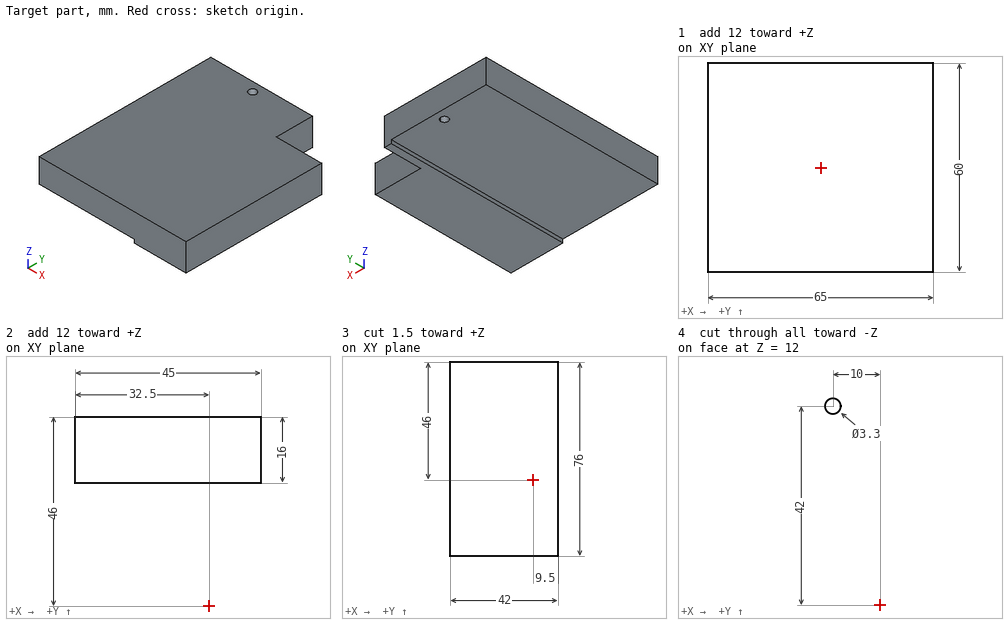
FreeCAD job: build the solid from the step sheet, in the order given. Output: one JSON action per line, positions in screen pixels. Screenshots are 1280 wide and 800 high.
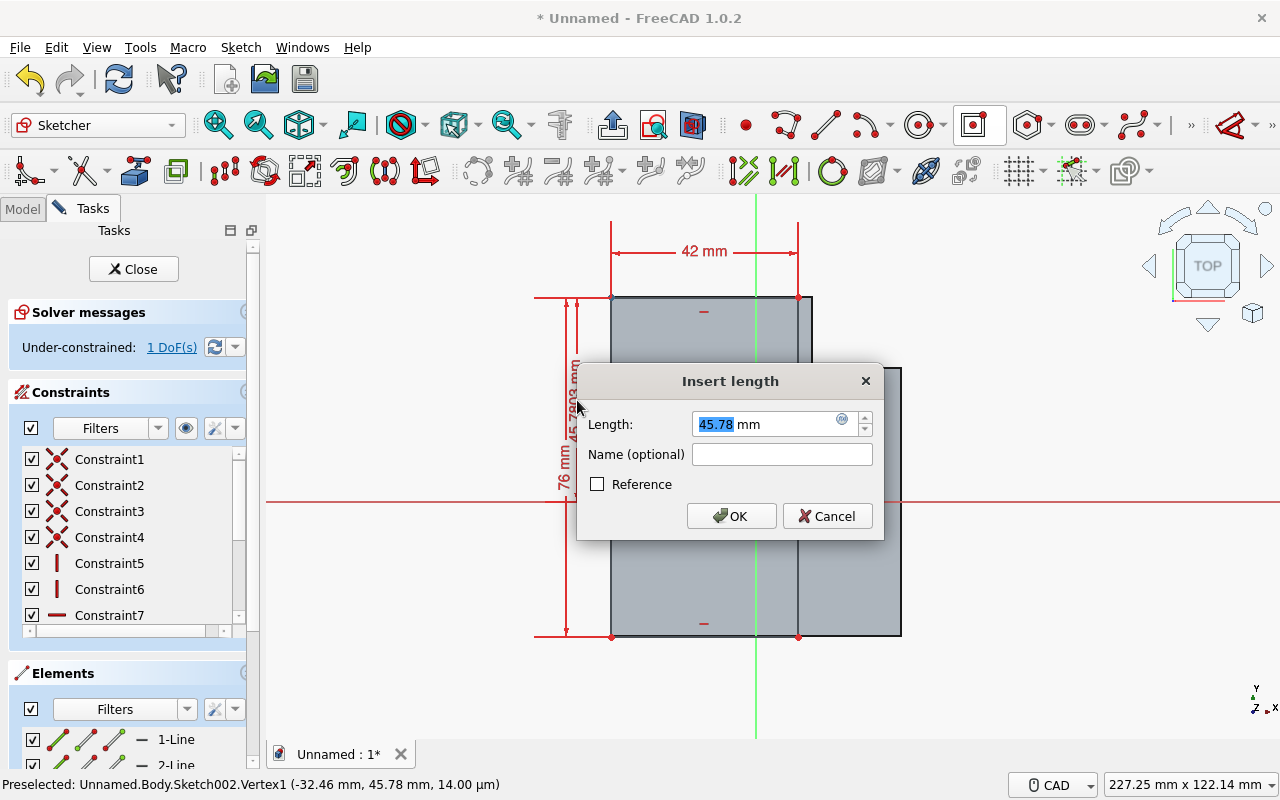
{"action": "type", "text": "46"}
{"action": "key", "text": "Return"}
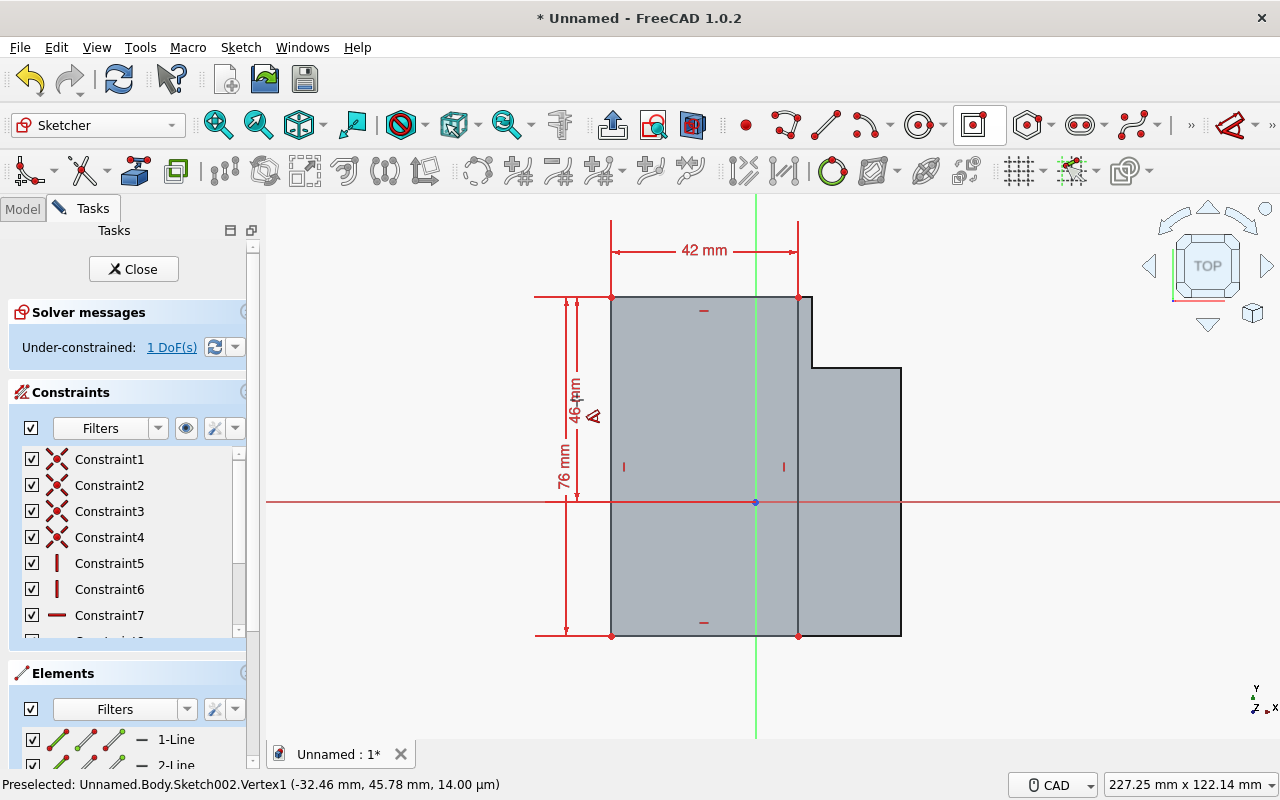
{"action": "left_click", "coordinate": [798, 636]}
{"action": "left_click", "coordinate": [777, 670]}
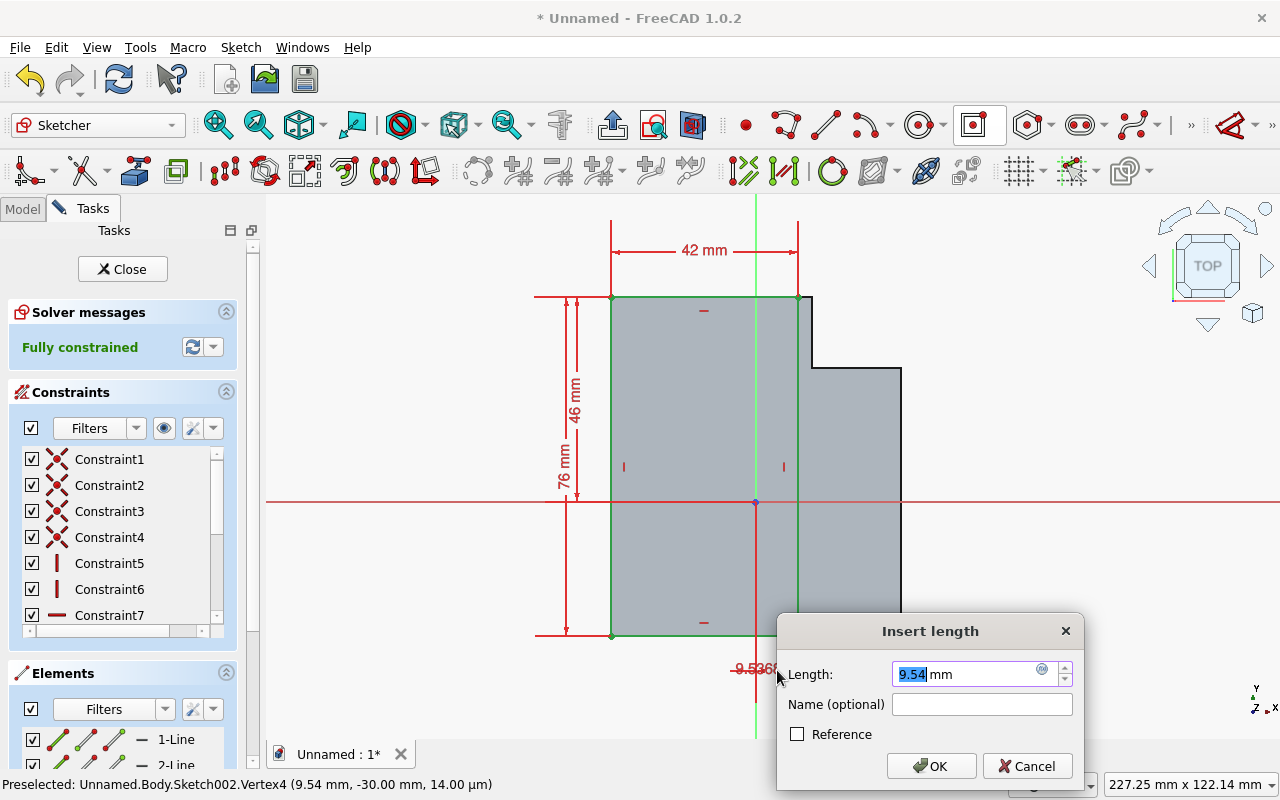
{"action": "type", "text": "9.5"}
{"action": "key", "text": "Return"}
{"action": "key", "text": "Escape"}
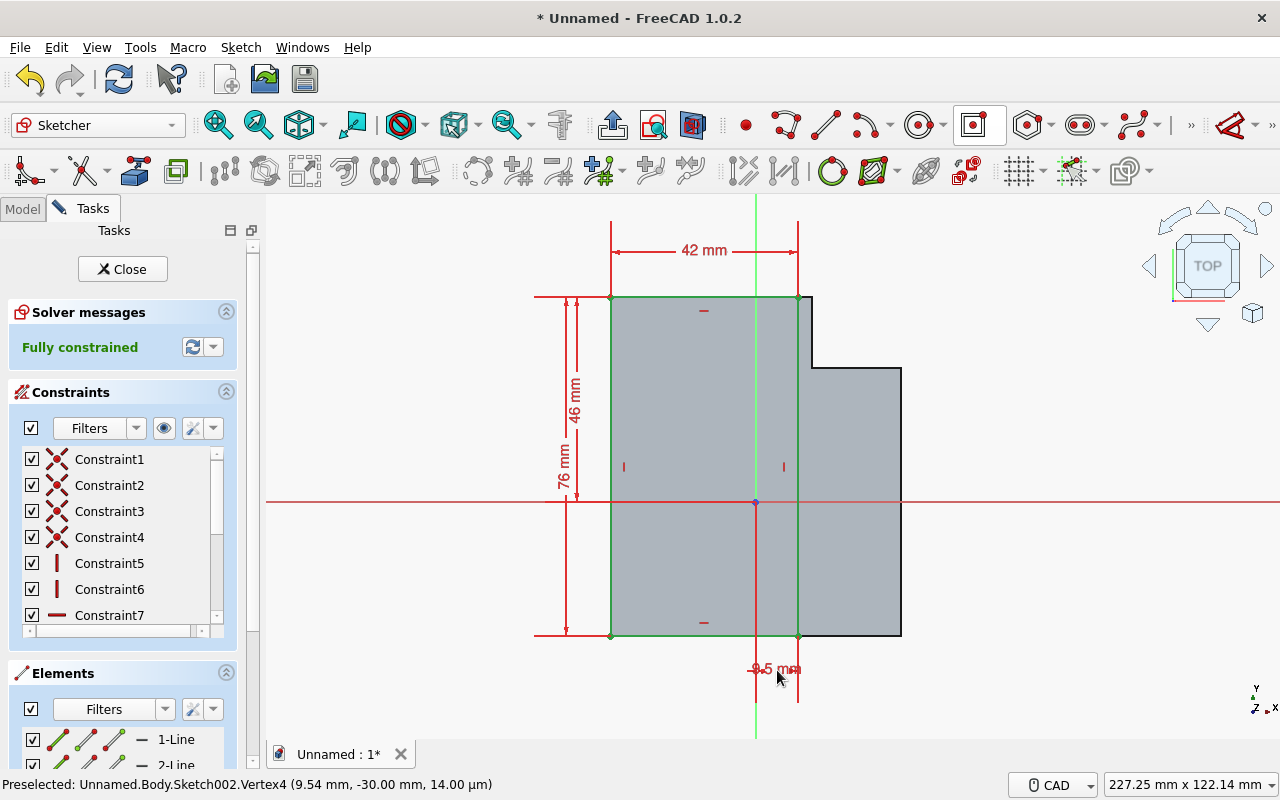
{"action": "left_click", "coordinate": [123, 269]}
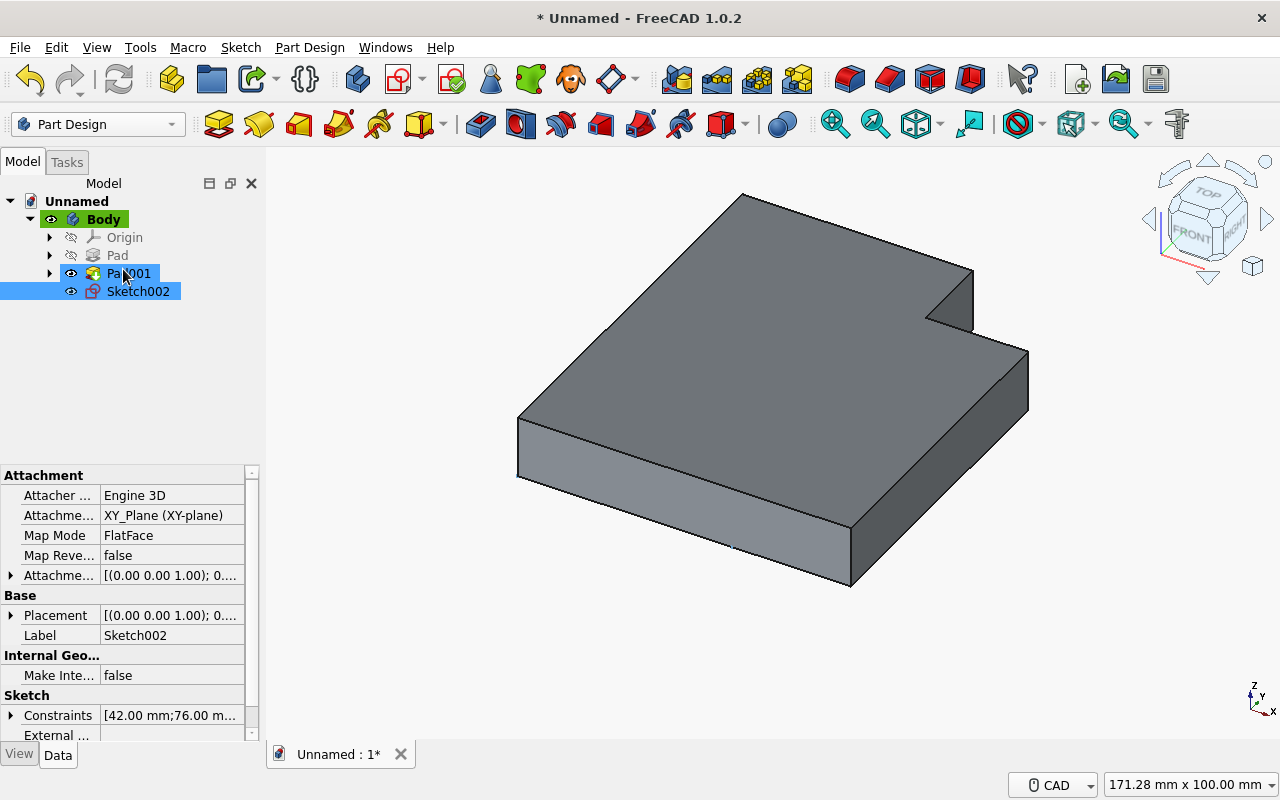
{"action": "left_click", "coordinate": [482, 124]}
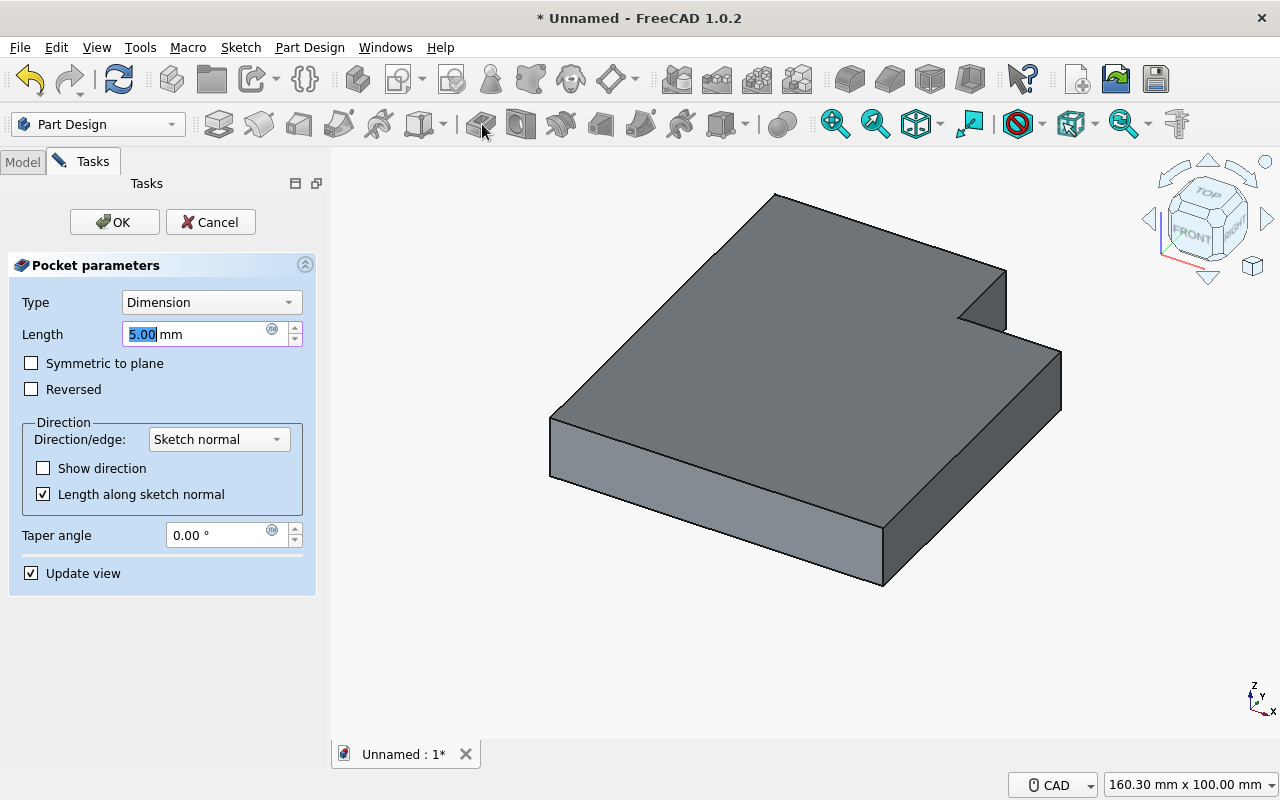
{"action": "type", "text": "1.5"}
{"action": "key", "text": "Tab"}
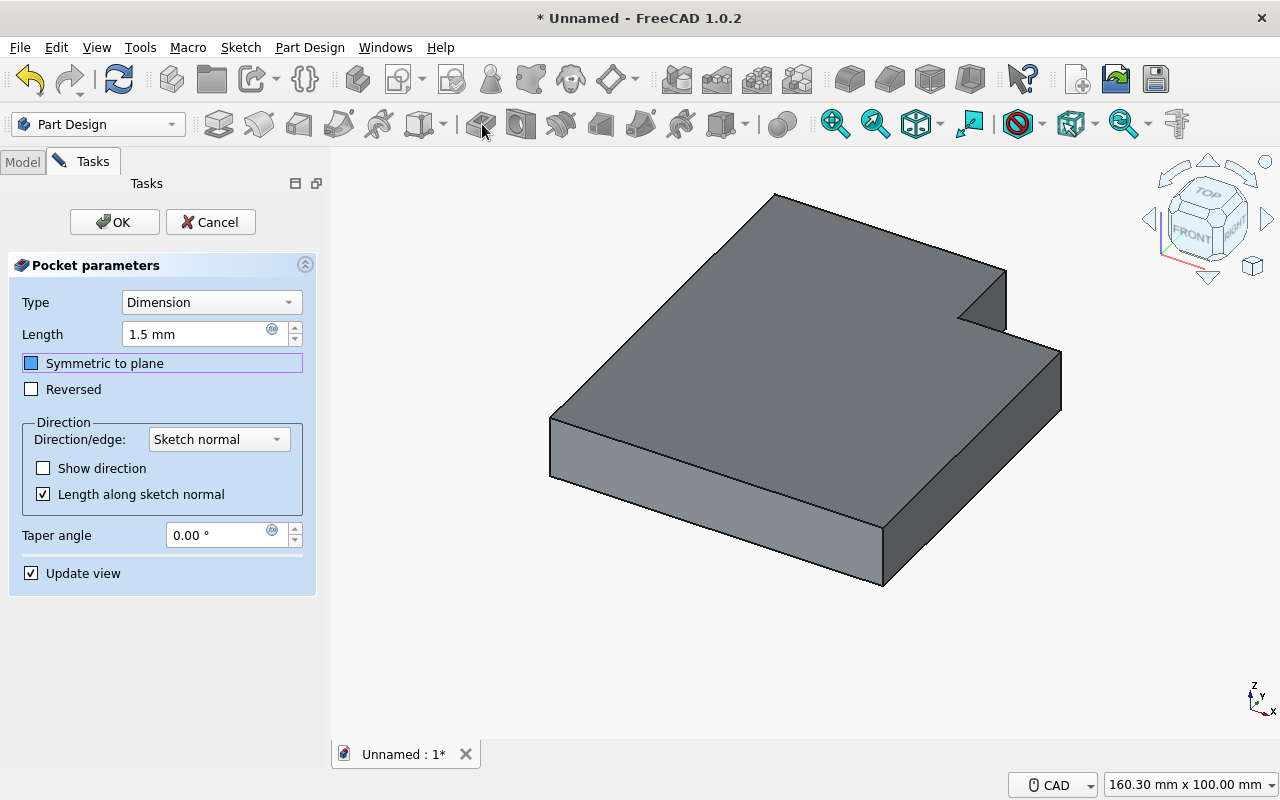
{"action": "left_click", "coordinate": [30, 389]}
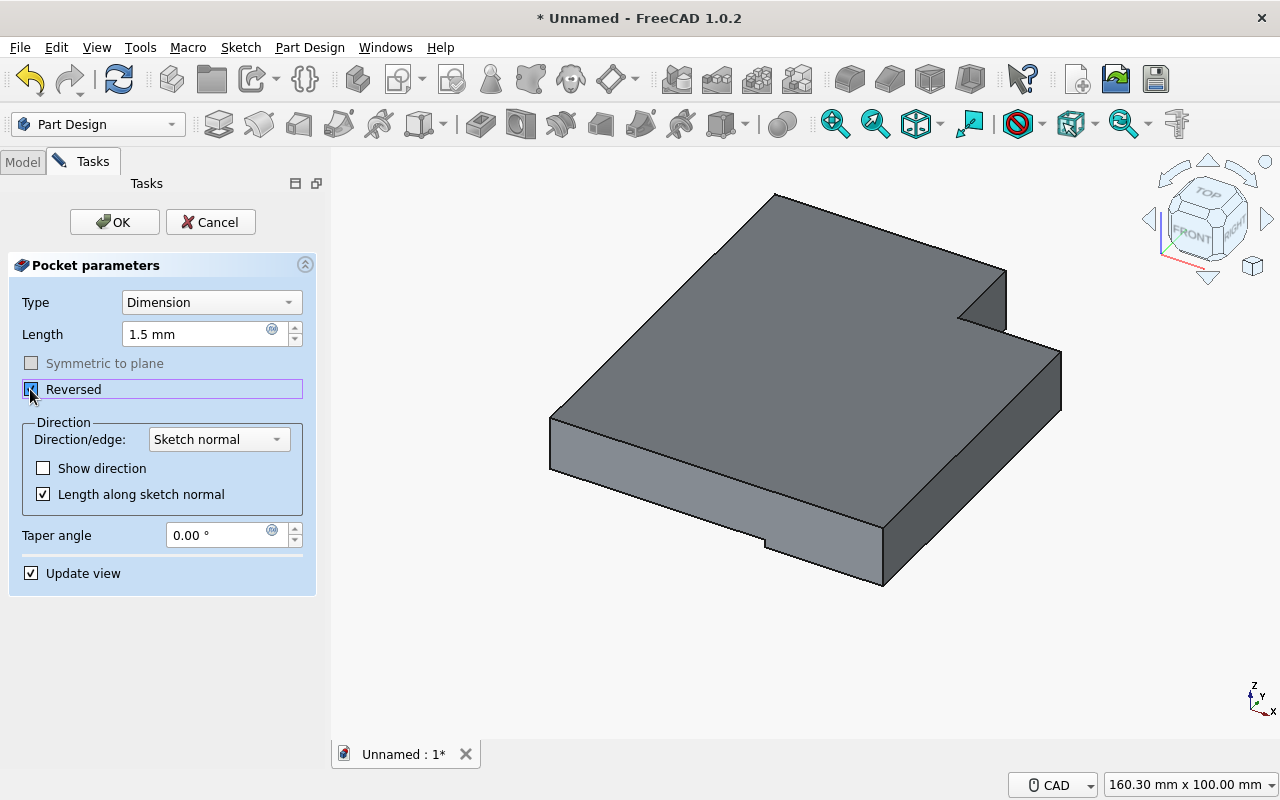
{"action": "left_click", "coordinate": [115, 222]}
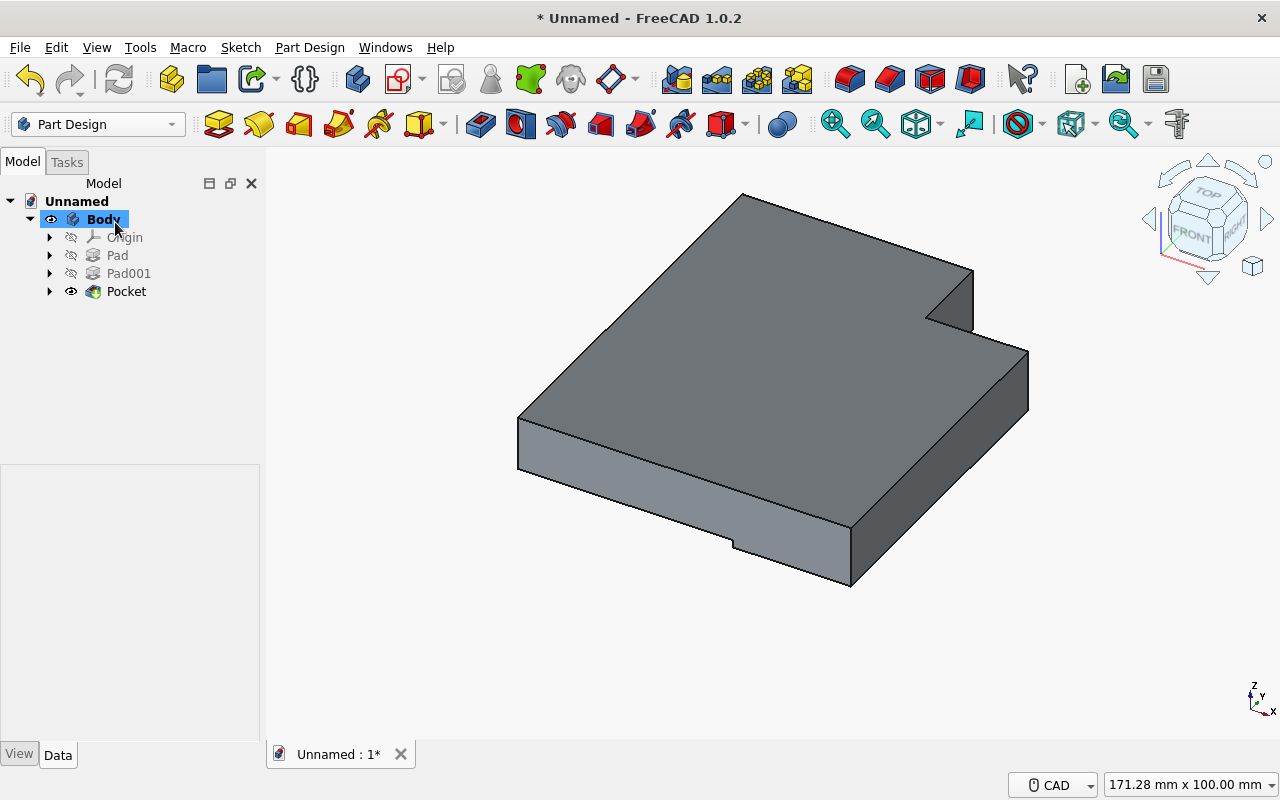
{"action": "left_click", "coordinate": [765, 392]}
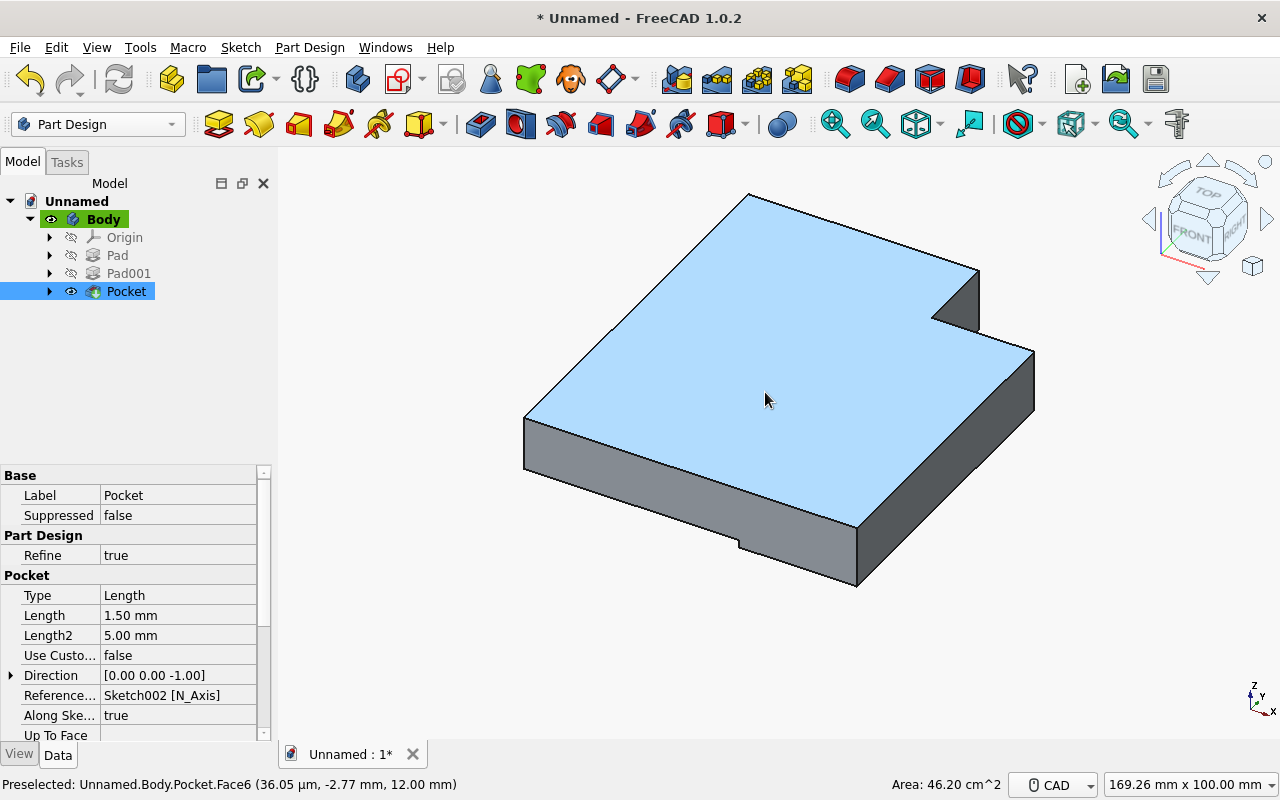
{"action": "left_click", "coordinate": [398, 80]}